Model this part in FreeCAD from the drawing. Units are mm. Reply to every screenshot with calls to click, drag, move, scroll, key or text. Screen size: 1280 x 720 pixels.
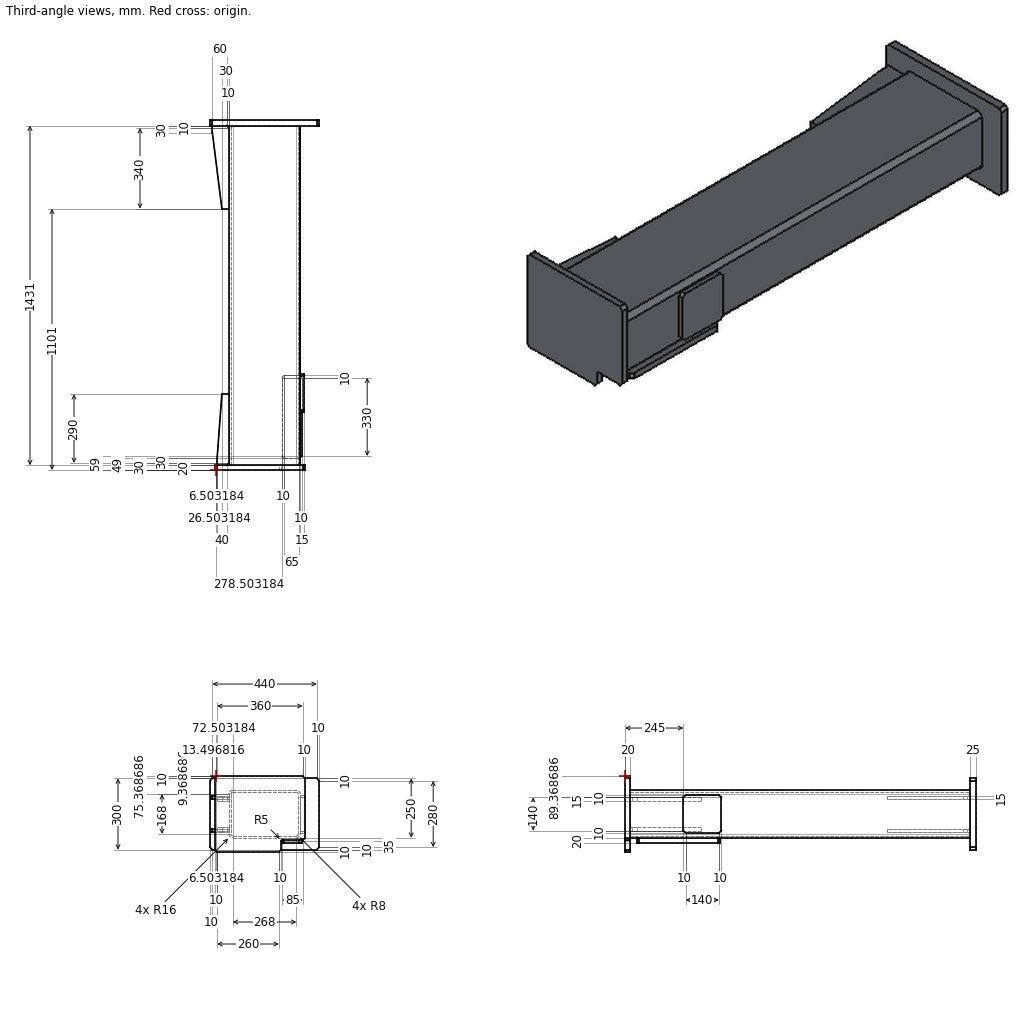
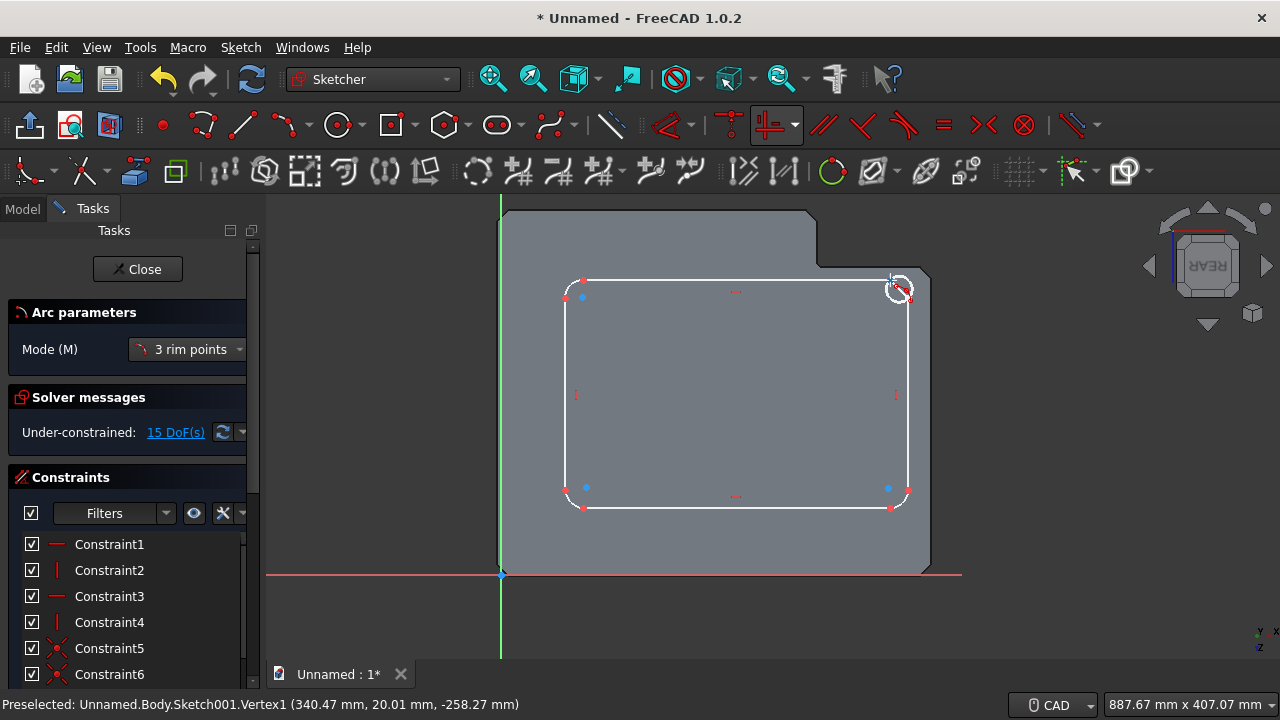
scroll(903, 284, up, 6)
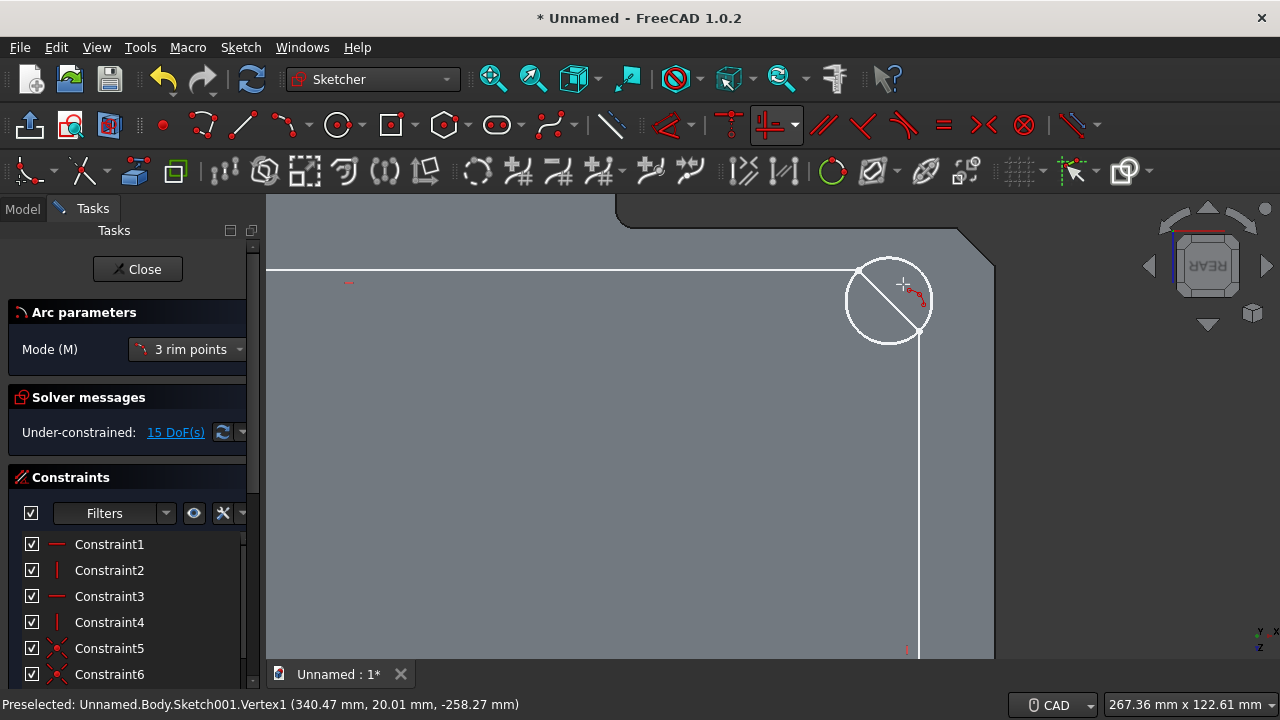
click(902, 284)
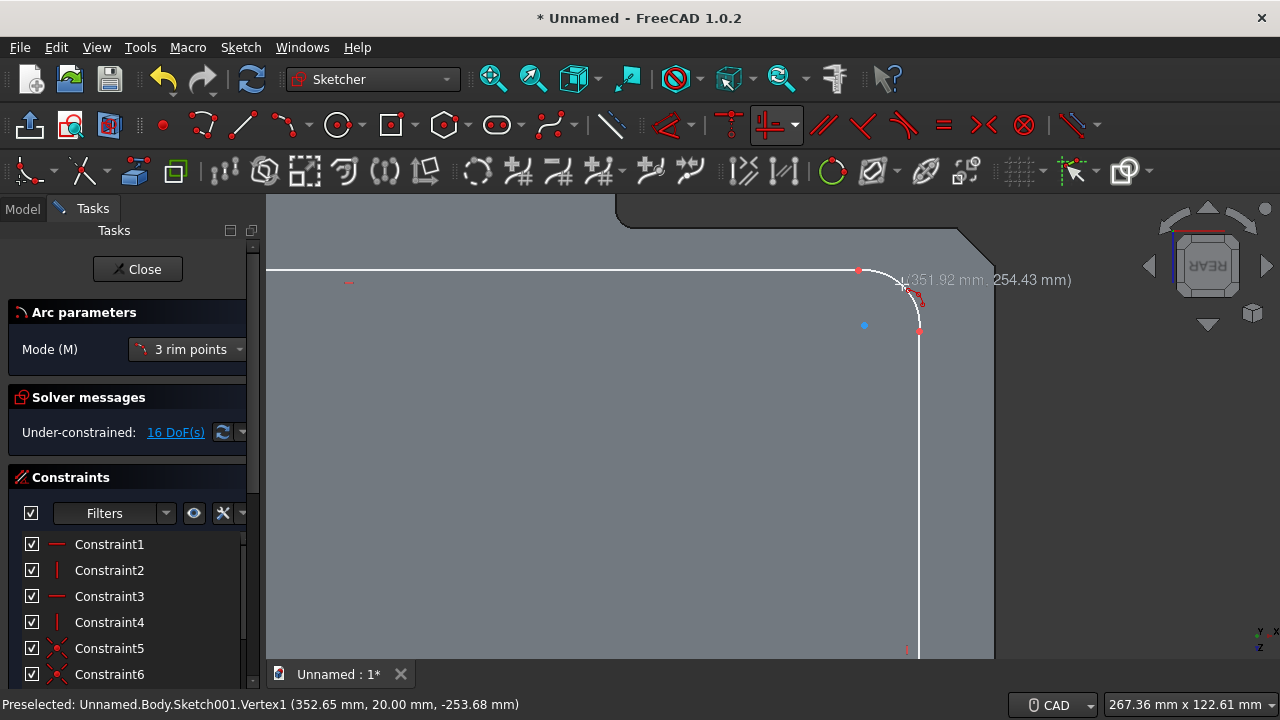
click(244, 126)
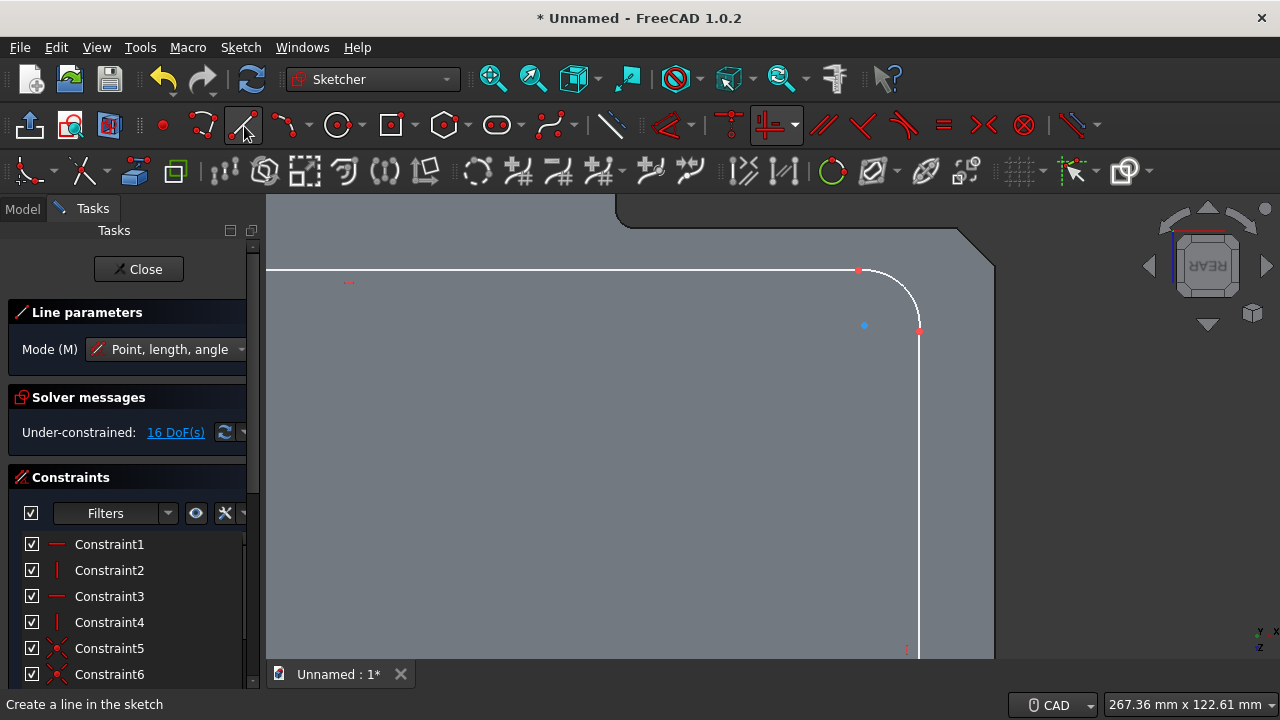
scroll(903, 284, down, 6)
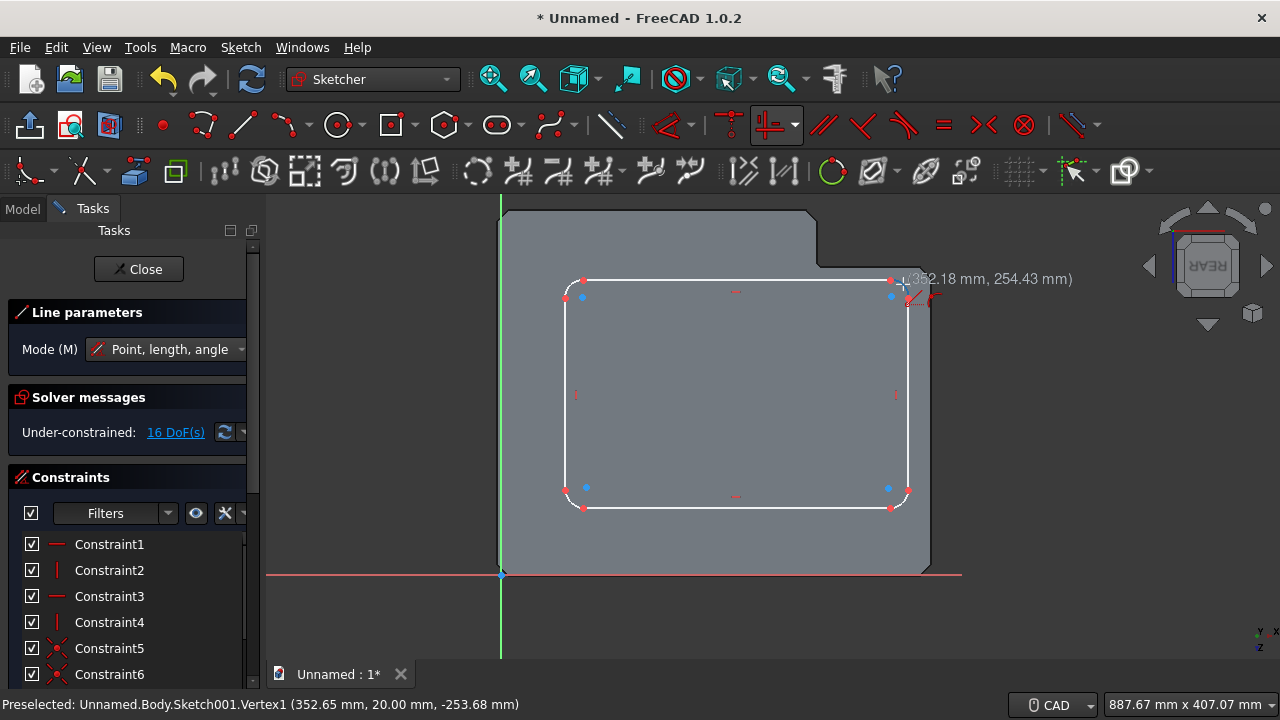
scroll(584, 288, up, 3)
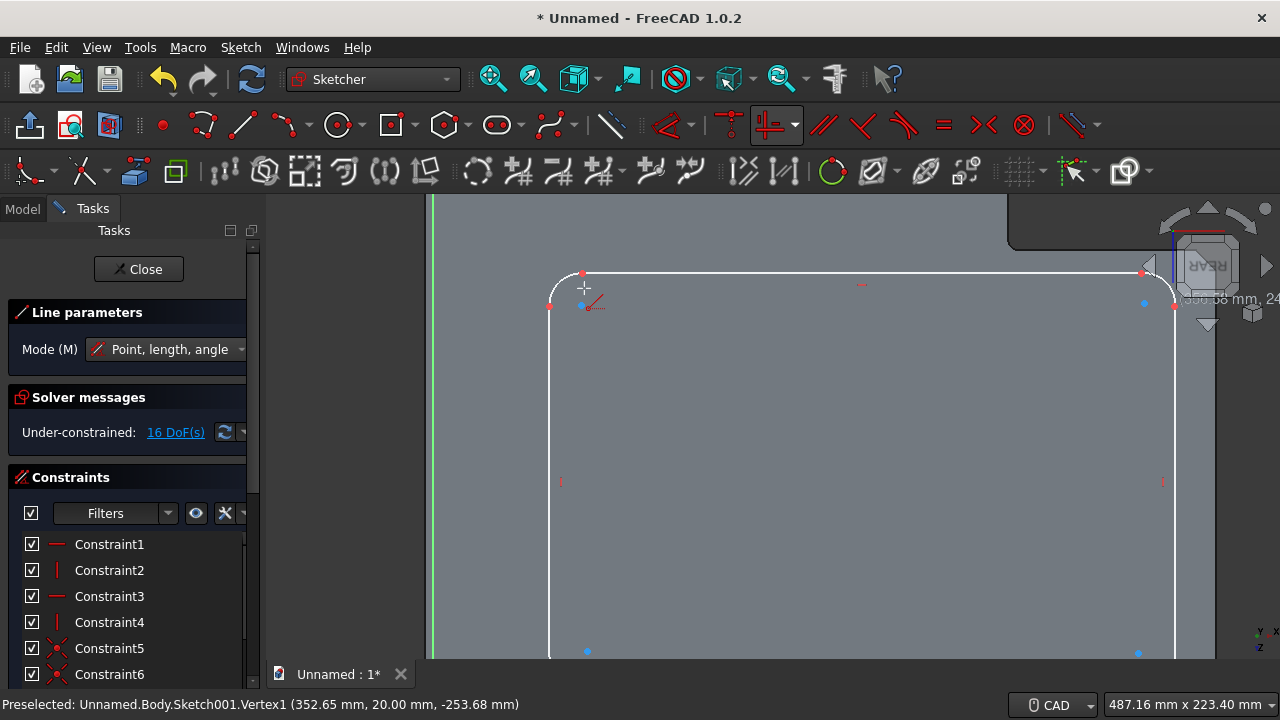
click(584, 288)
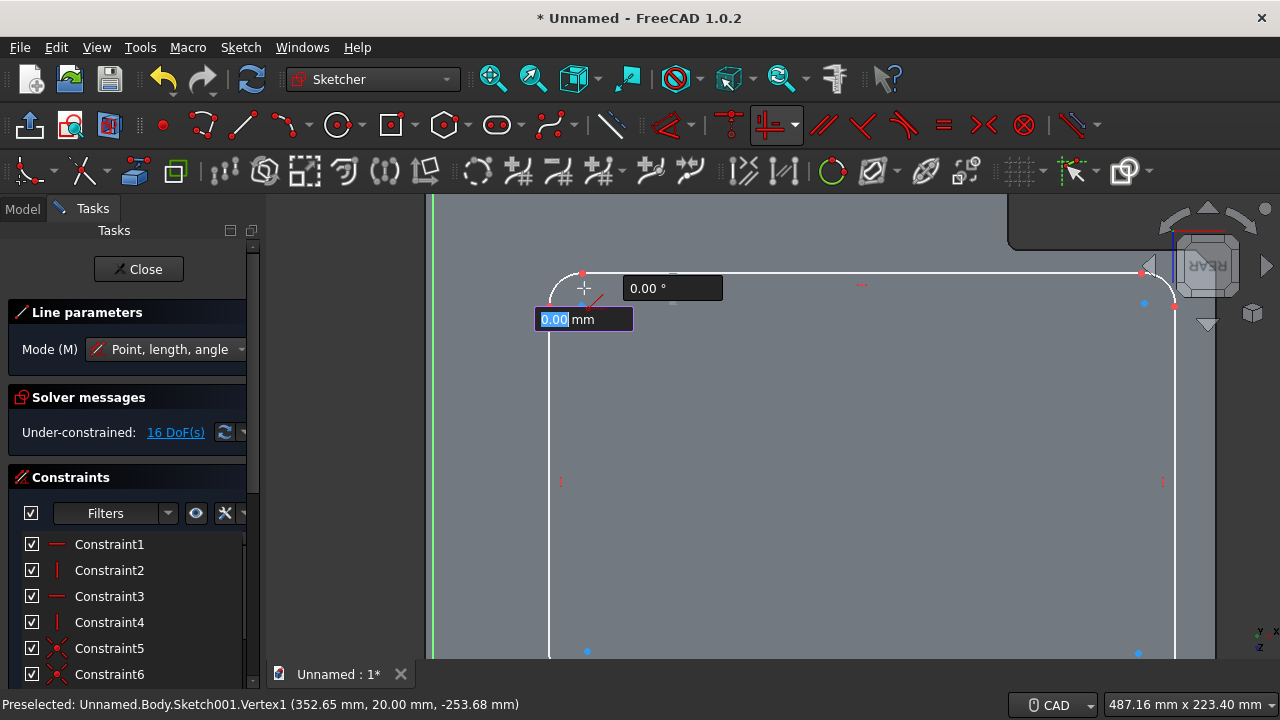
scroll(584, 287, down, 3)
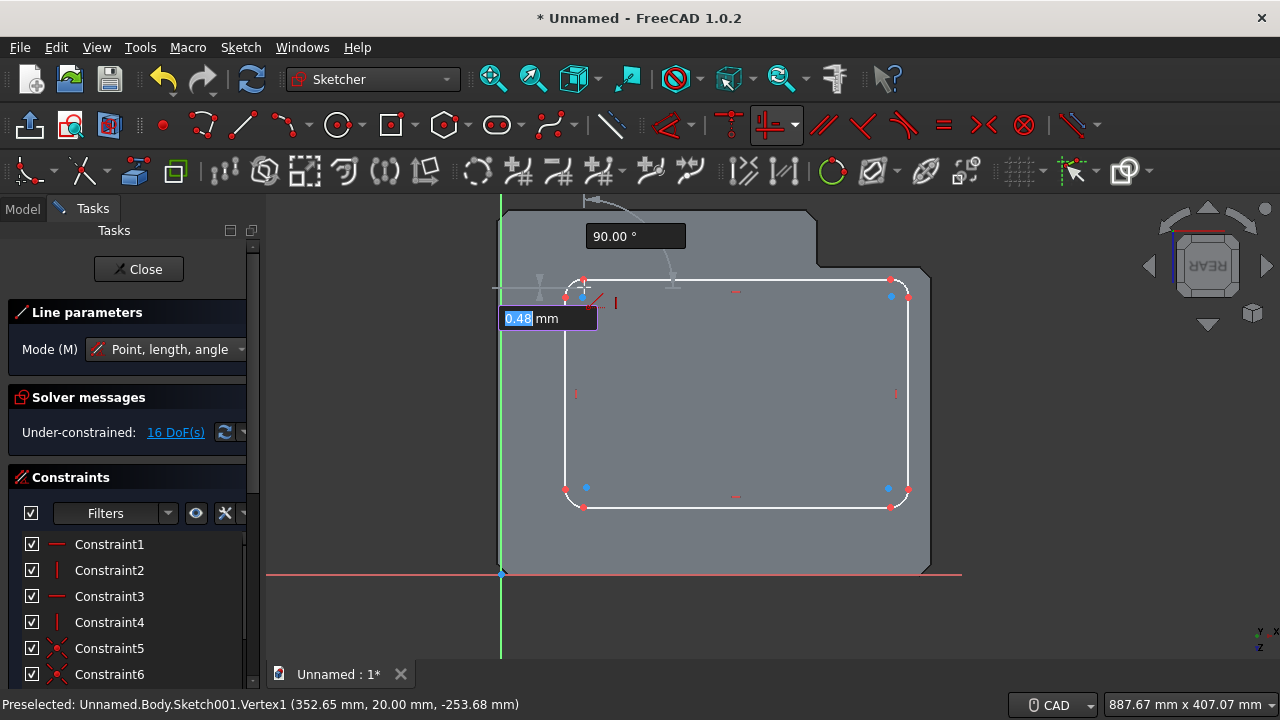
scroll(890, 287, up, 3)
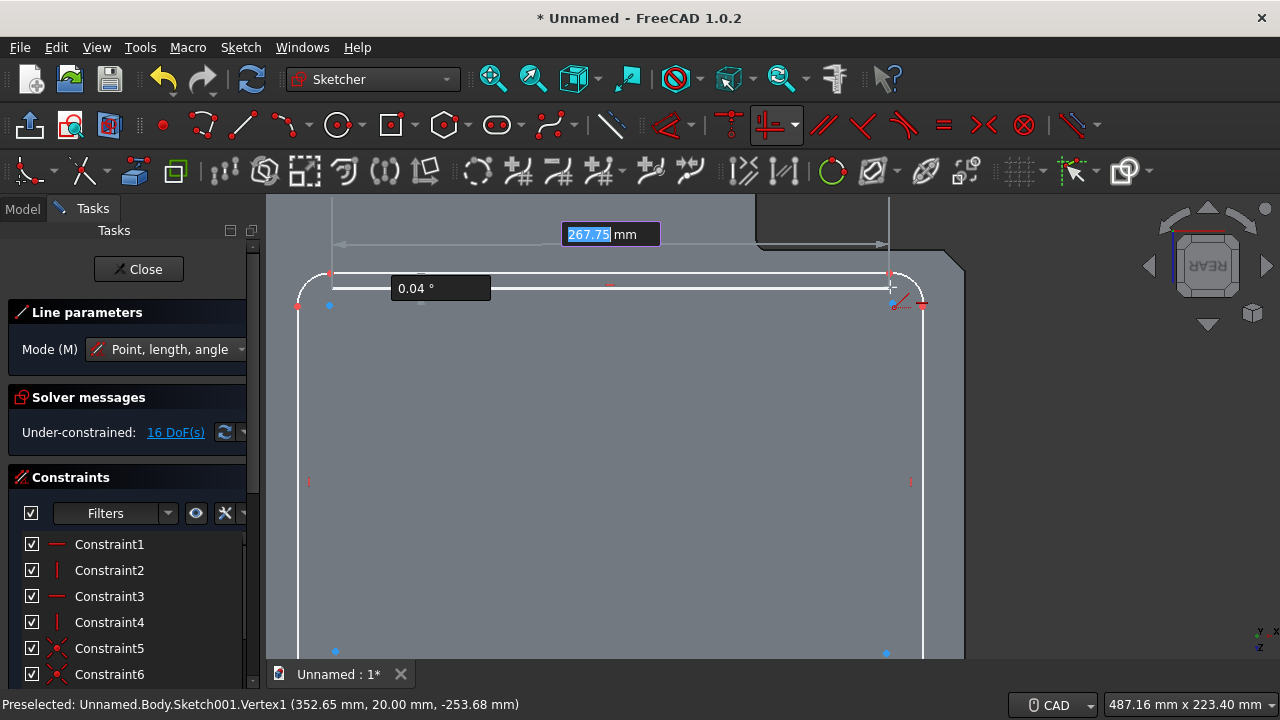
click(890, 288)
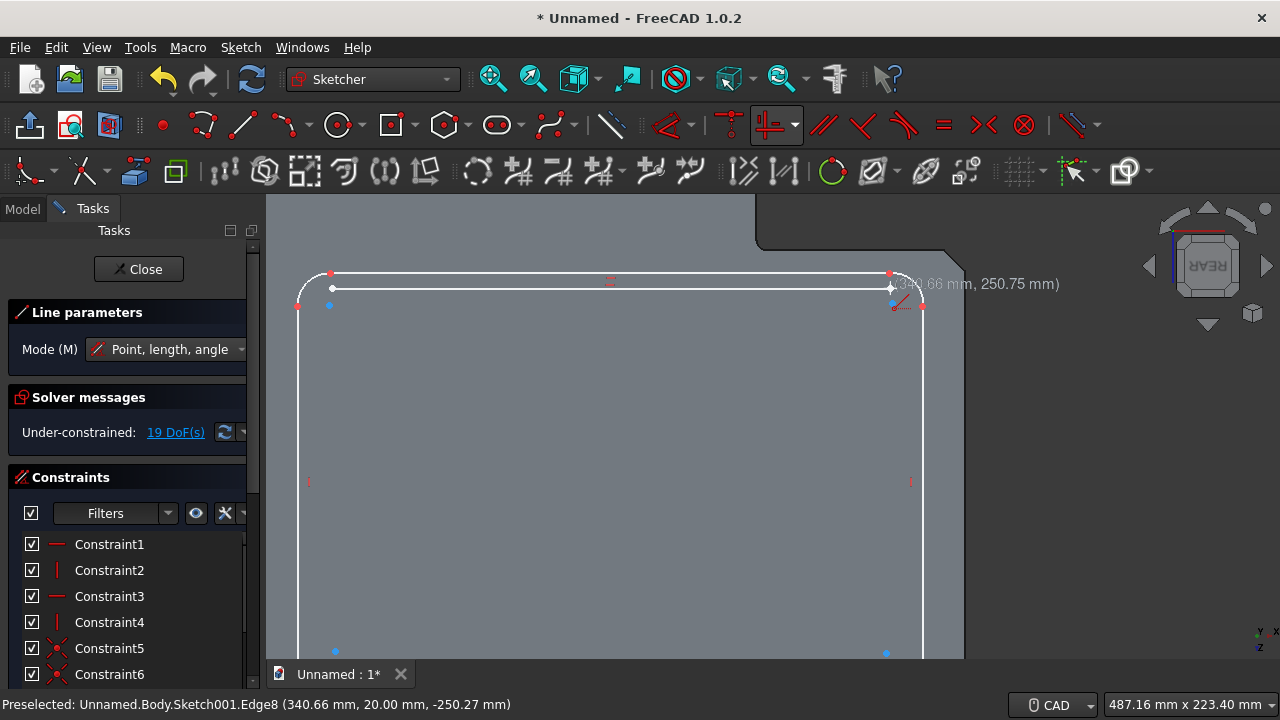
click(906, 304)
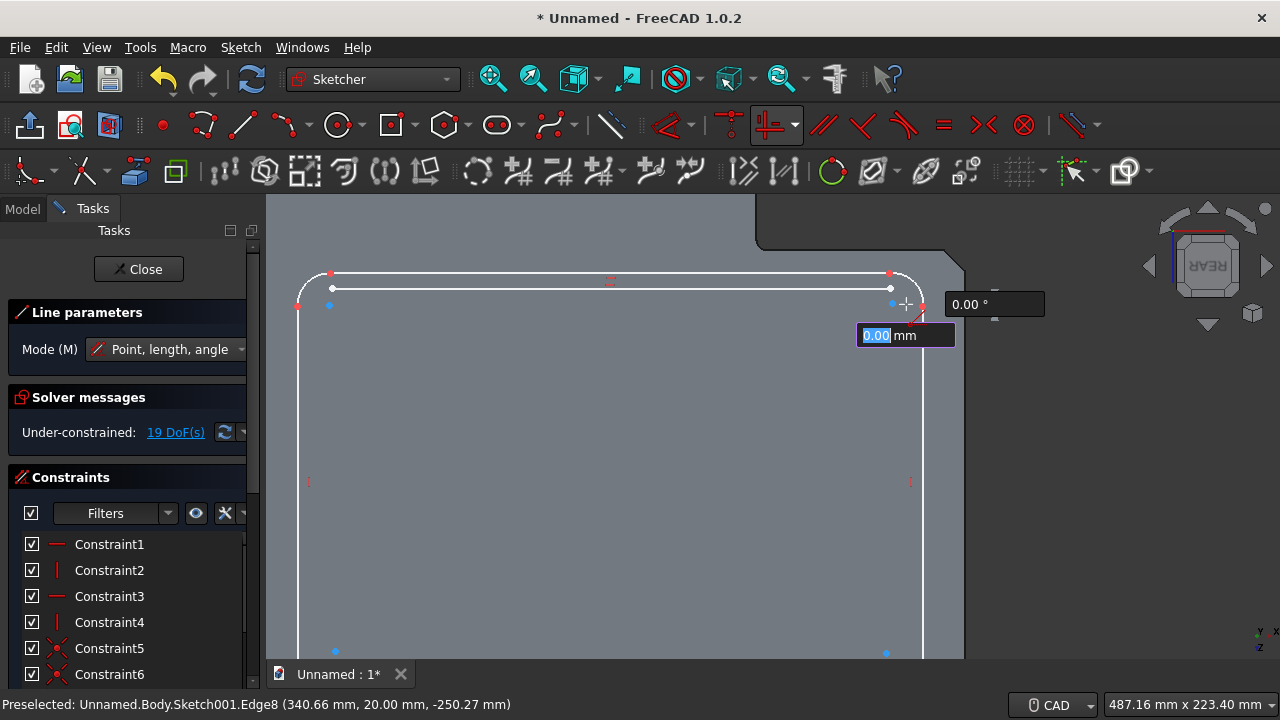
scroll(890, 287, down, 3)